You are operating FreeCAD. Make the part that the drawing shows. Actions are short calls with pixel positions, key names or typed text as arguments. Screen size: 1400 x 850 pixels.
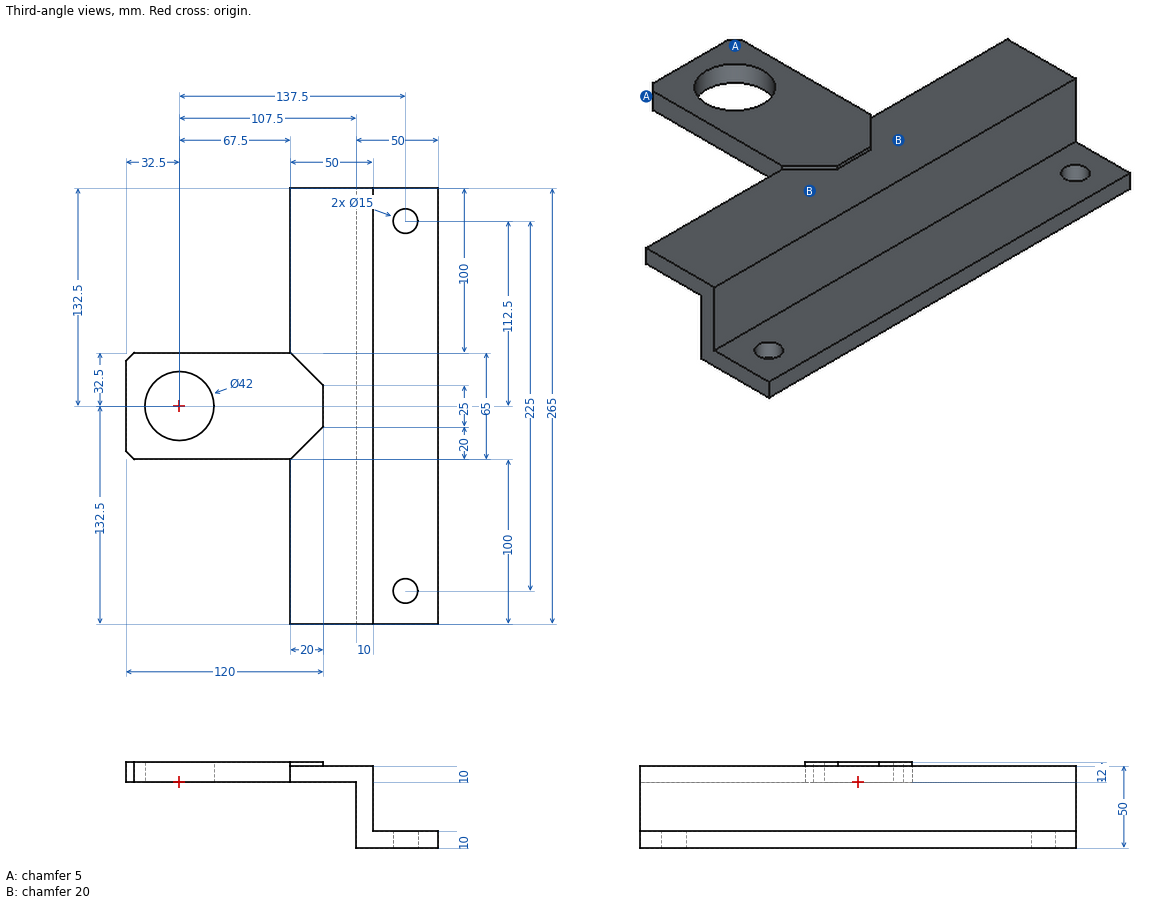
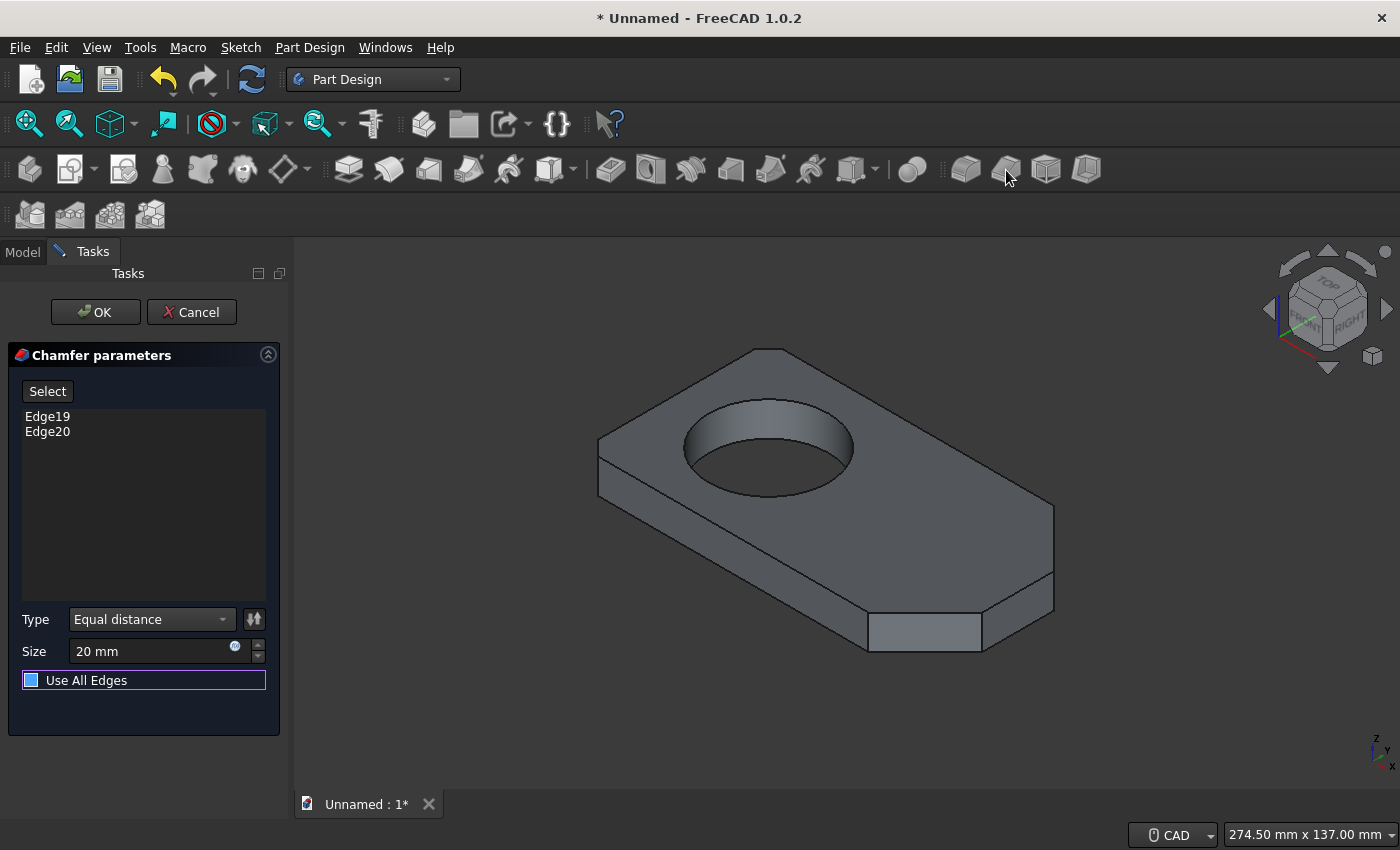
click(96, 312)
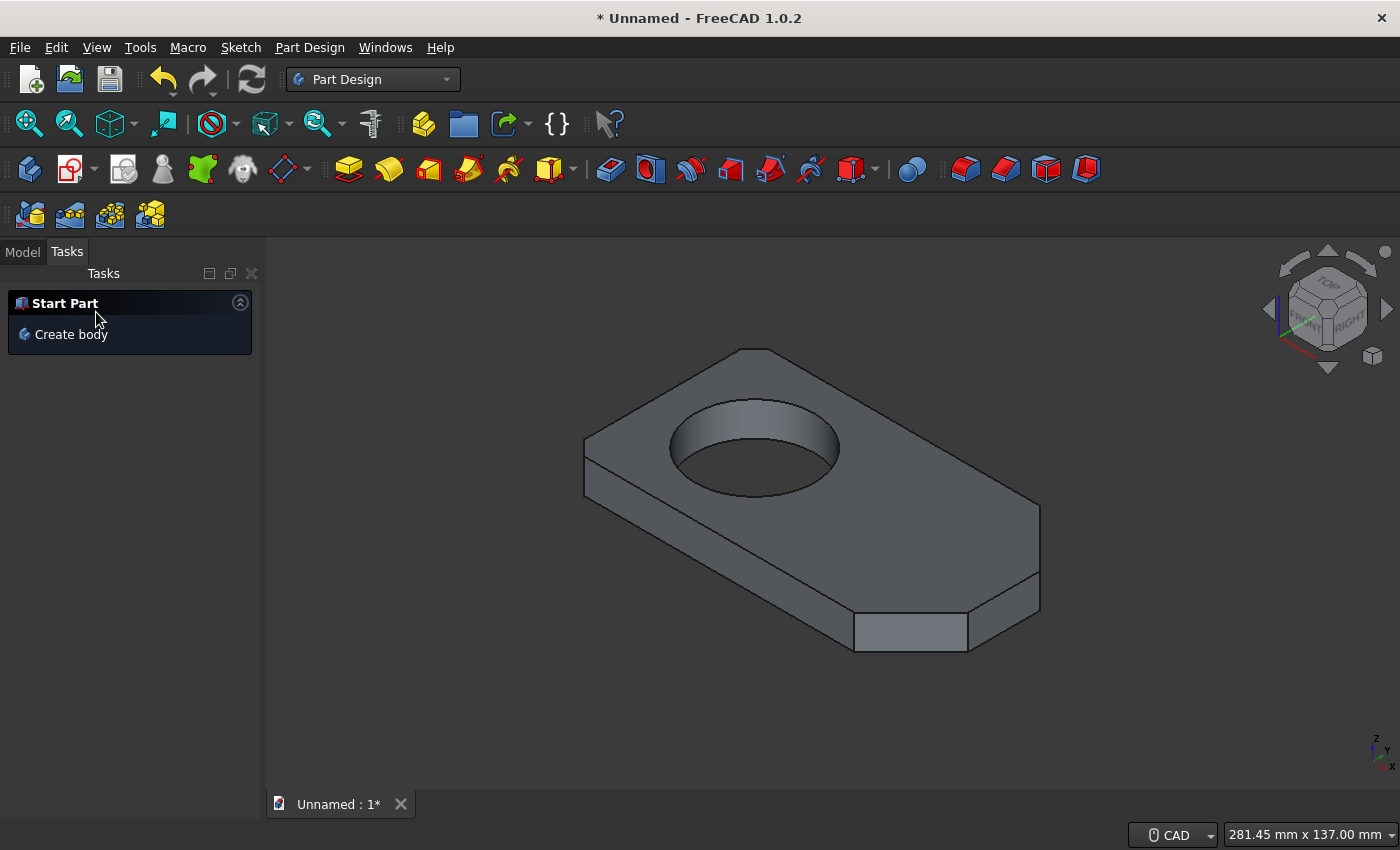
key(5)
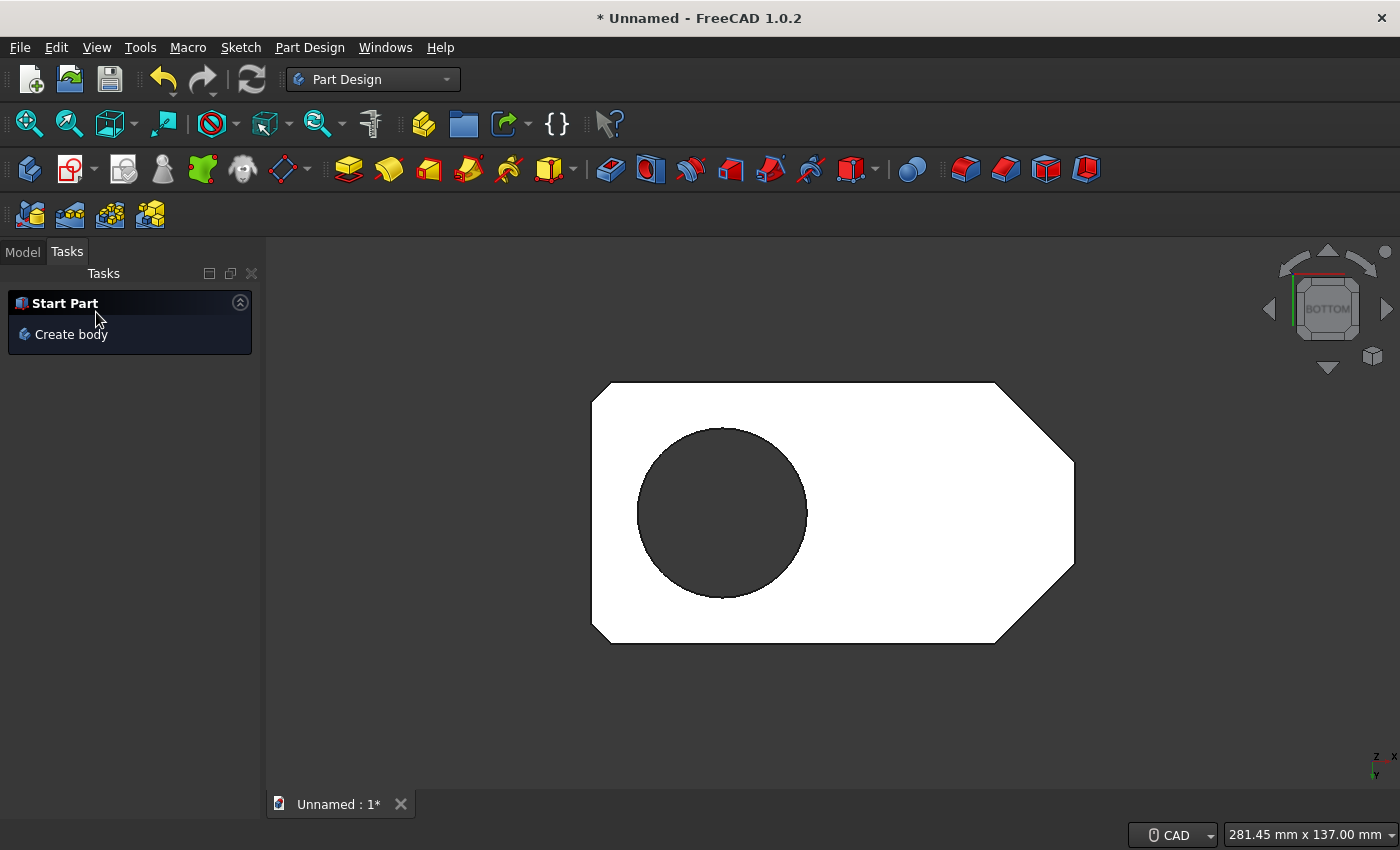
click(971, 512)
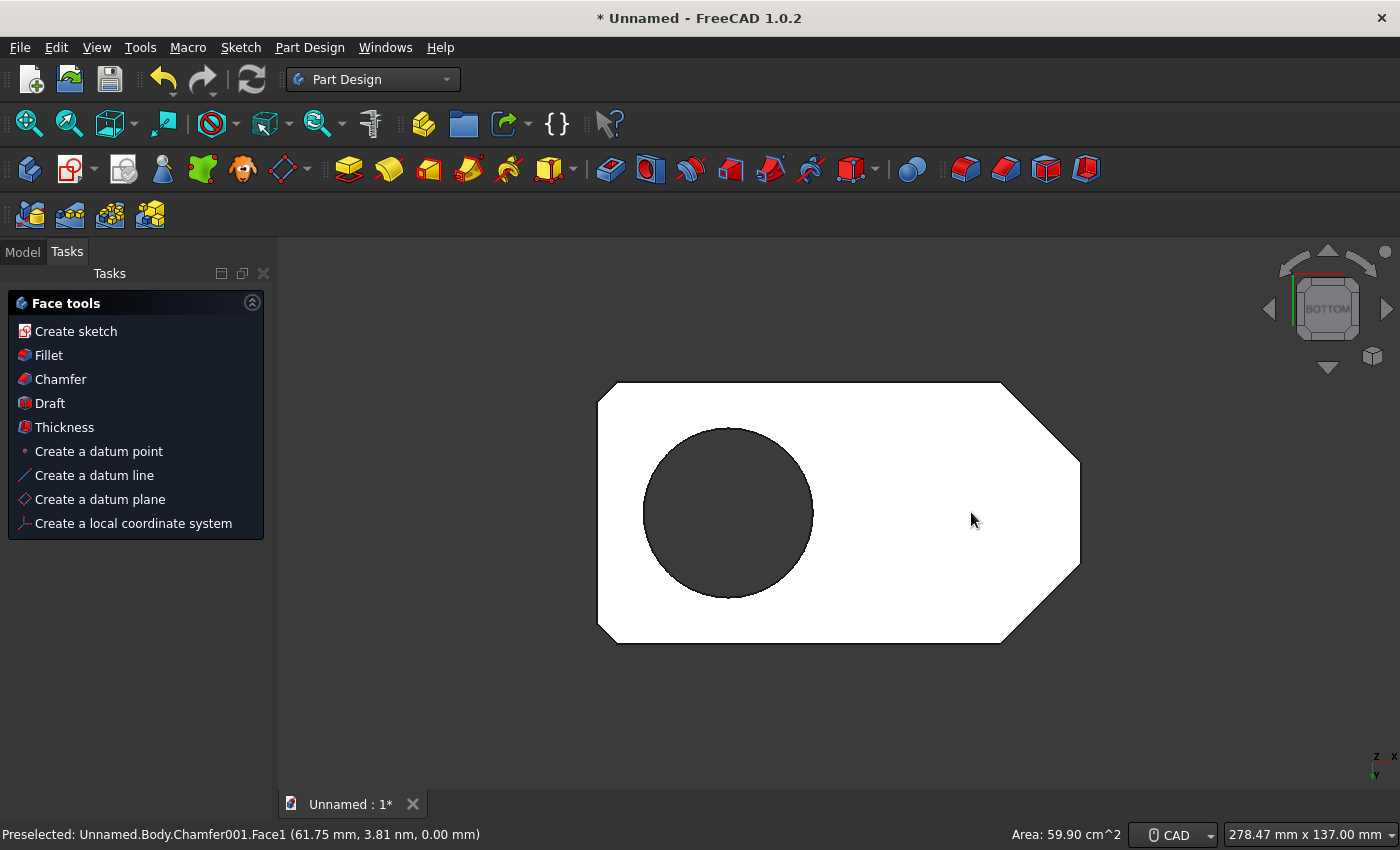
click(70, 170)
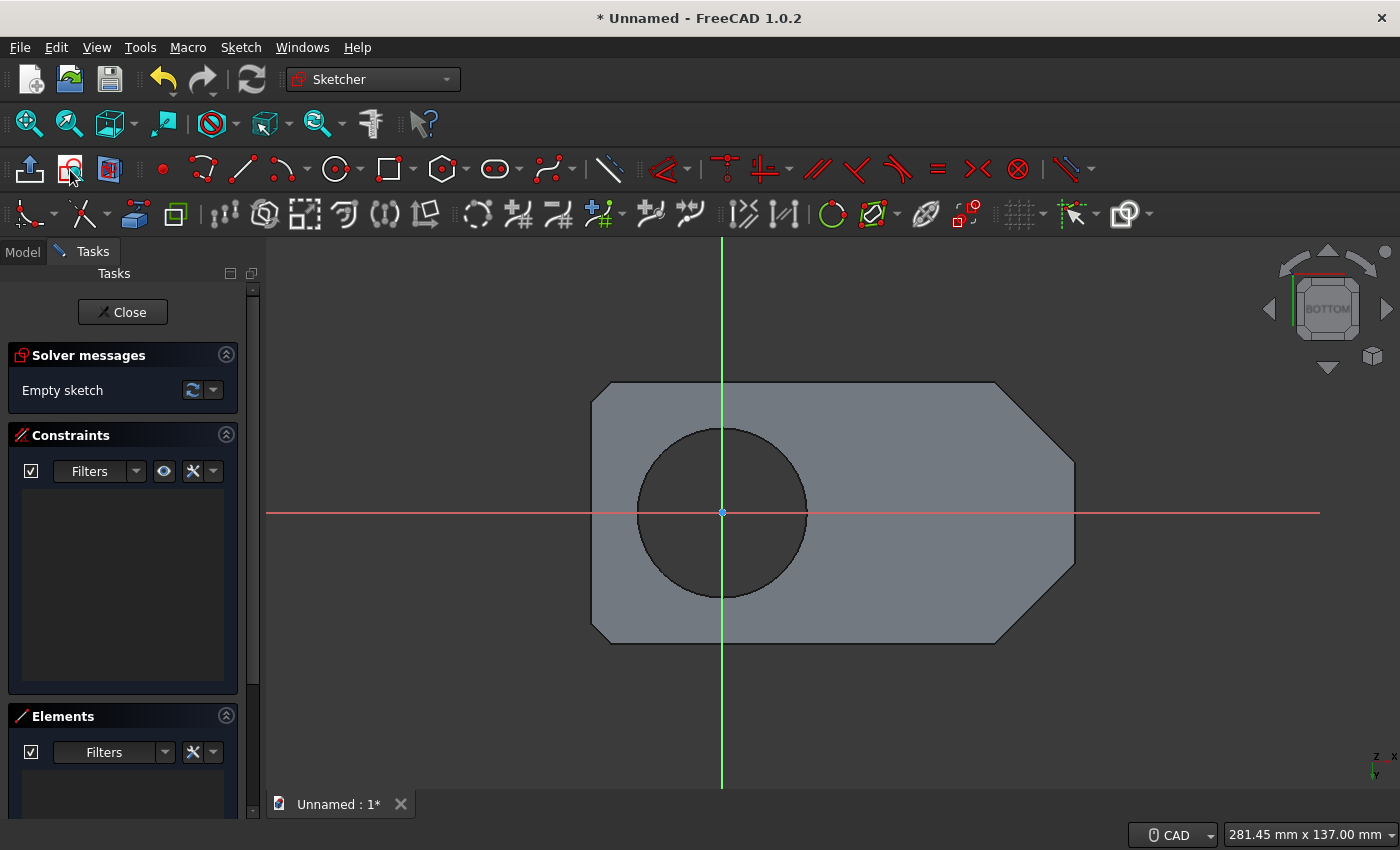
scroll(681, 513, down, 6)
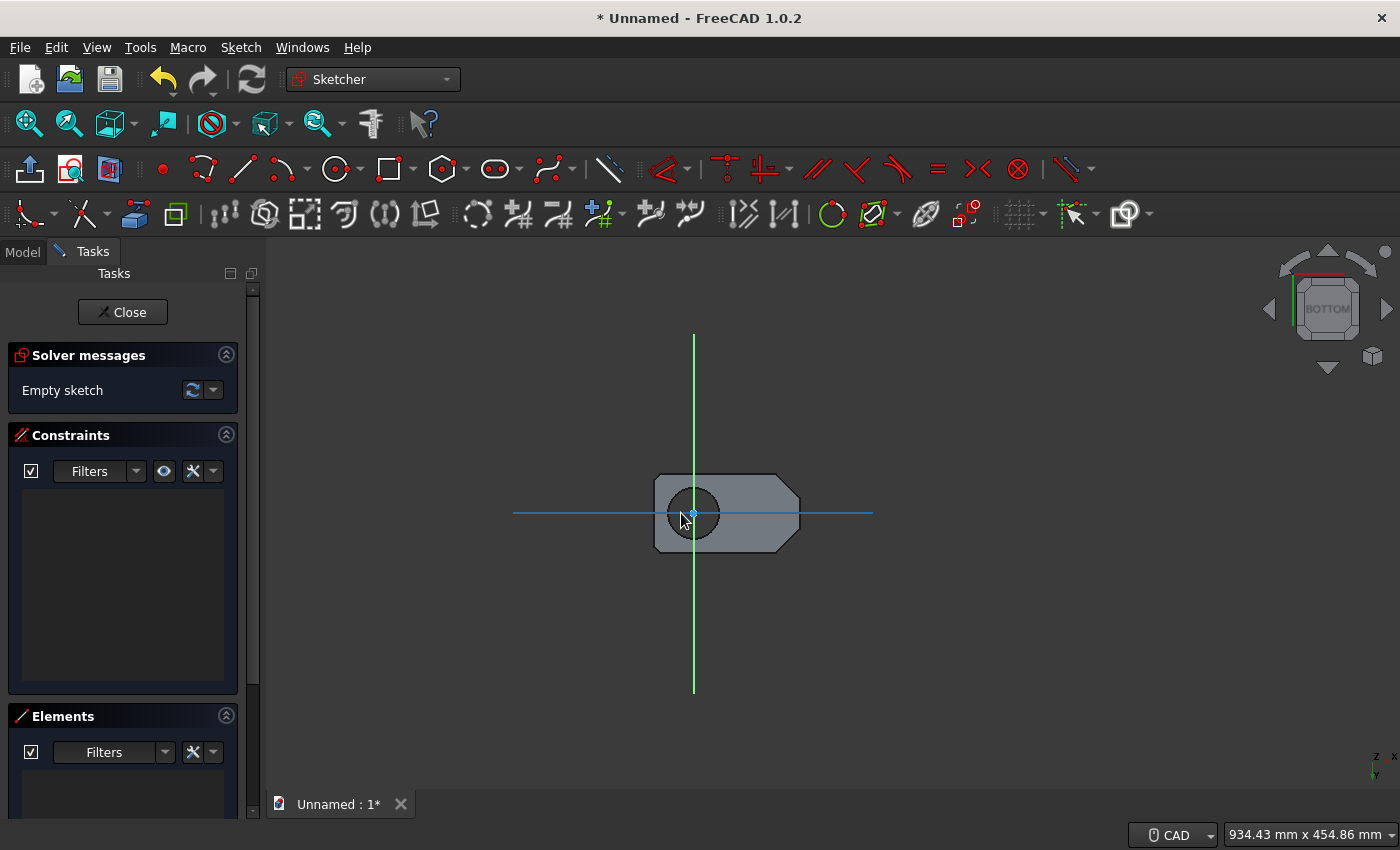
key(g)
key(m)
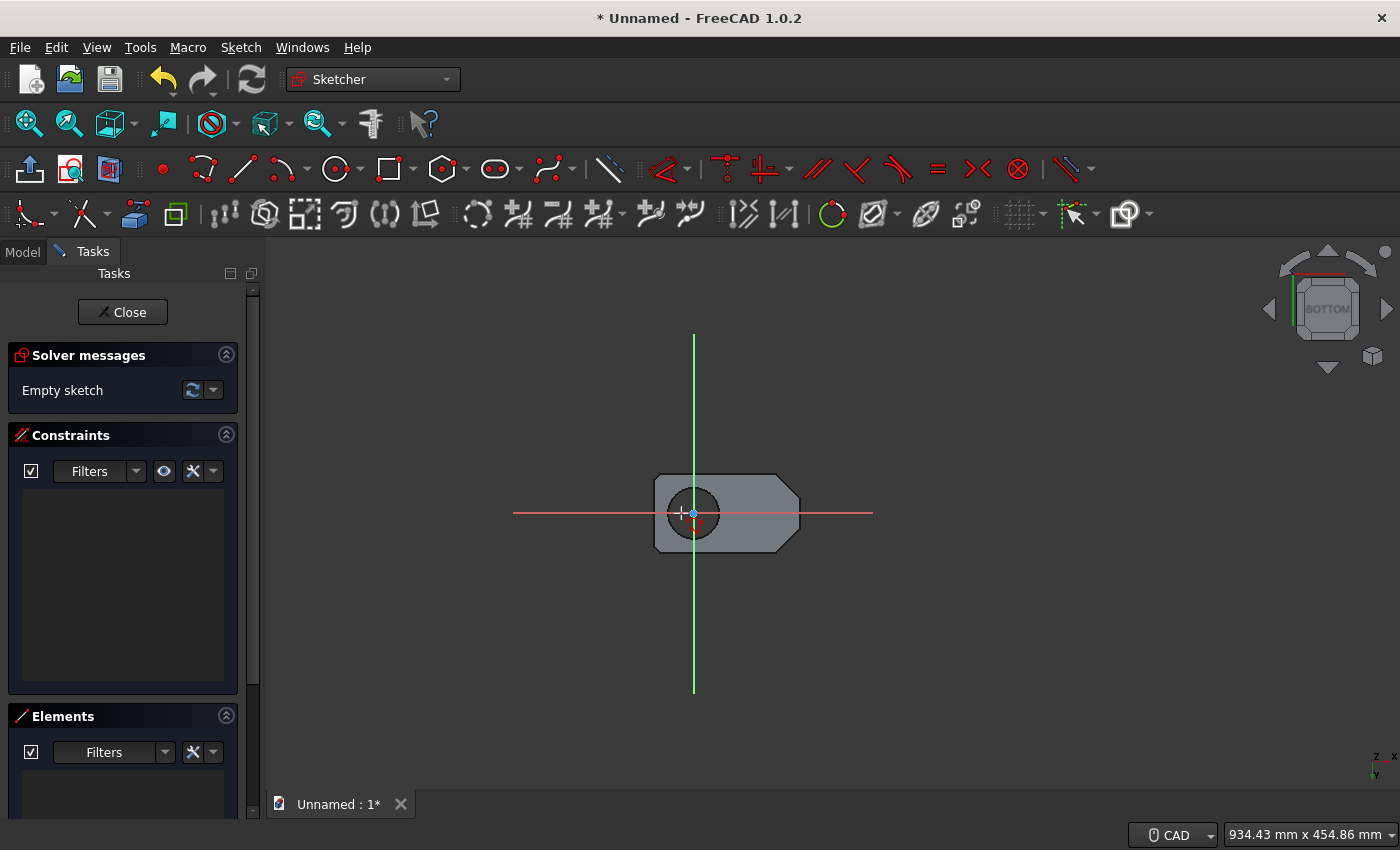
click(776, 553)
click(776, 674)
click(836, 674)
click(836, 353)
click(776, 353)
click(776, 474)
click(800, 498)
click(800, 529)
click(776, 554)
key(Escape)
key(Escape)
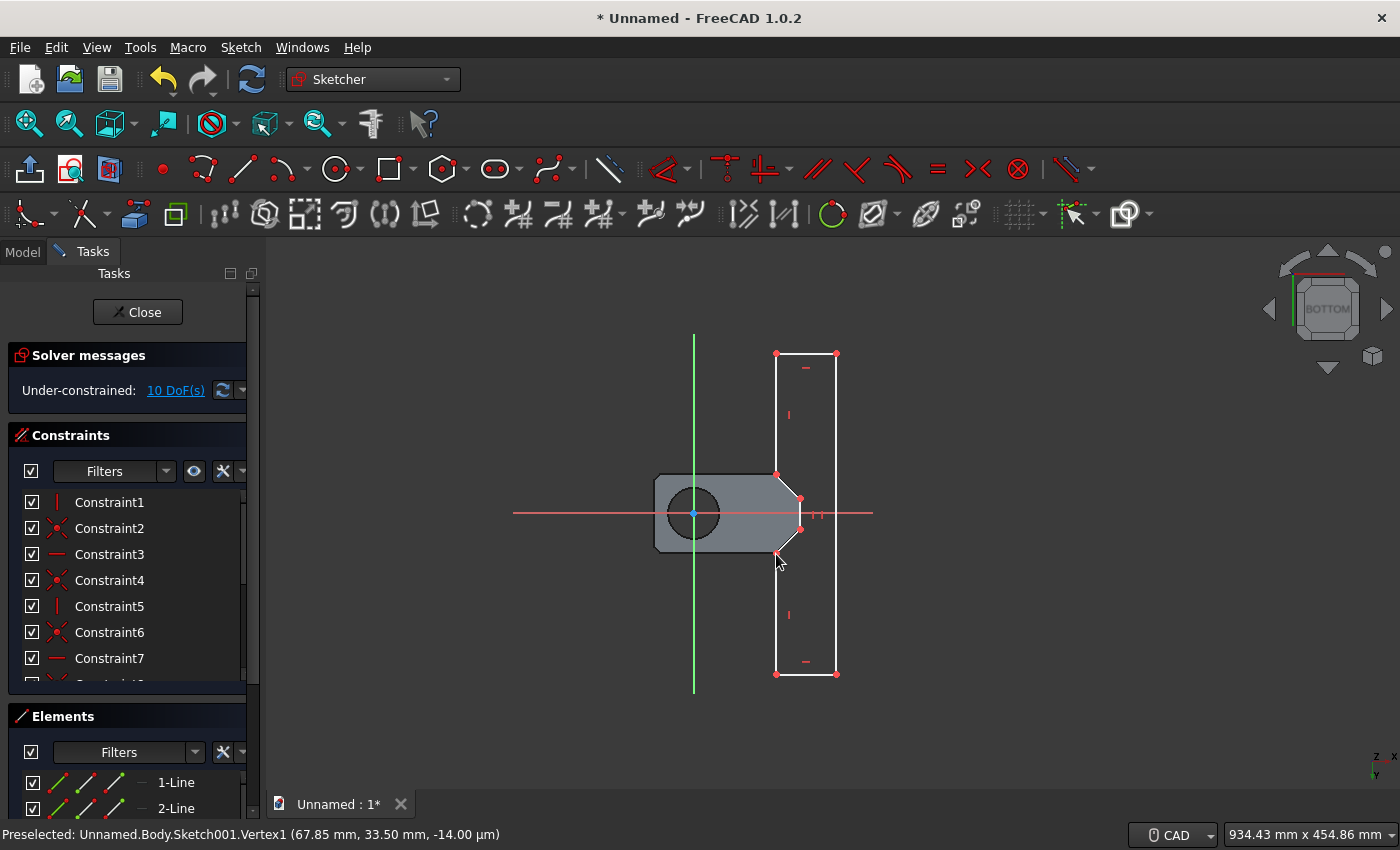
click(794, 675)